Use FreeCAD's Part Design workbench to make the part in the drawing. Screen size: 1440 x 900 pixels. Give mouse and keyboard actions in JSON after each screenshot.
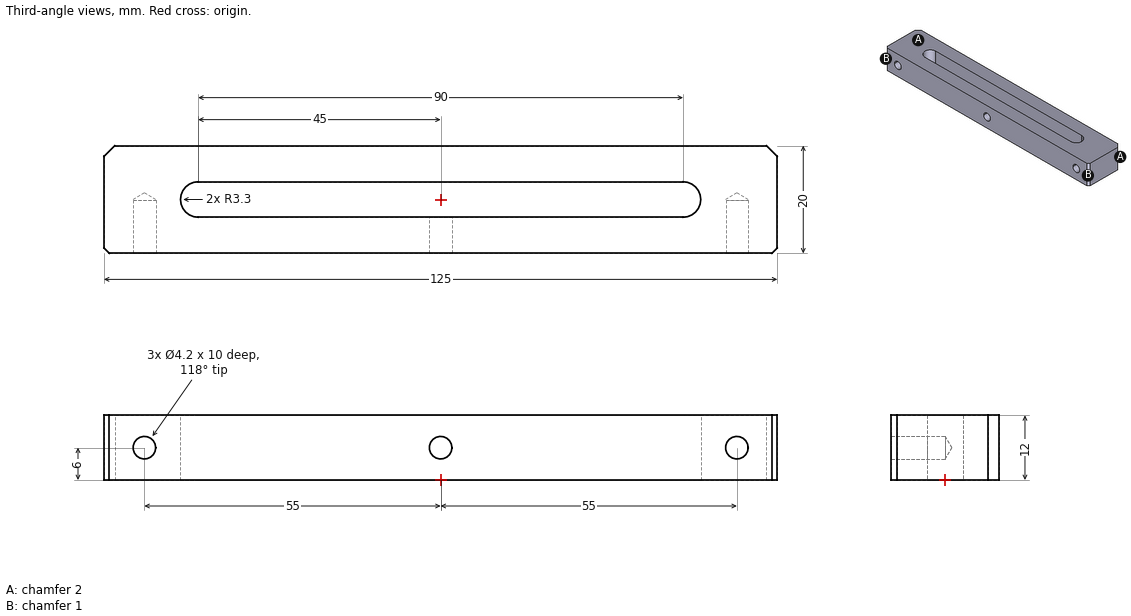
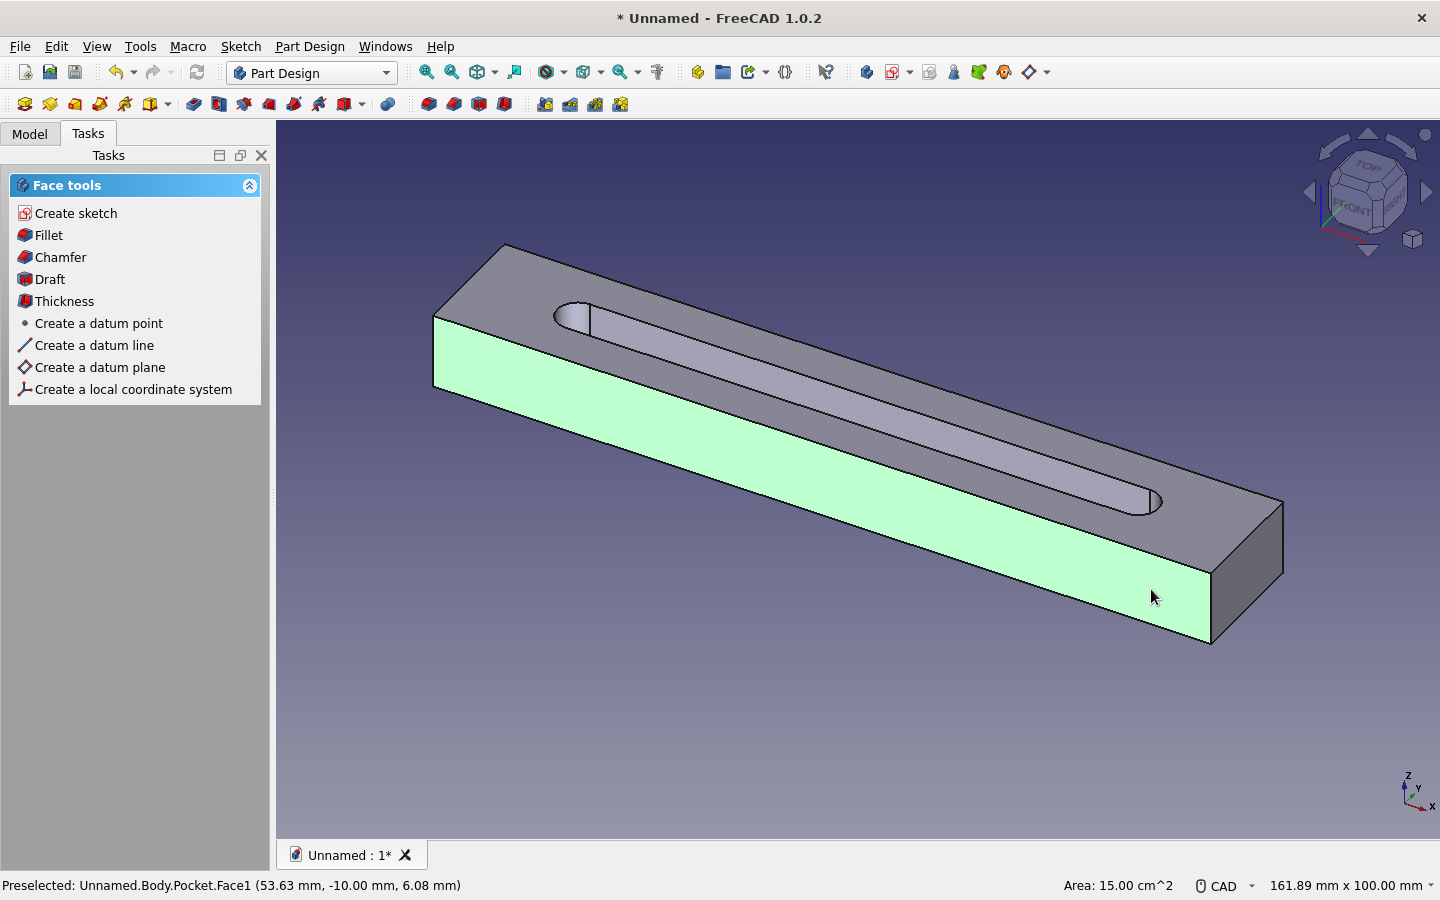
{"action": "left_click", "coordinate": [892, 72]}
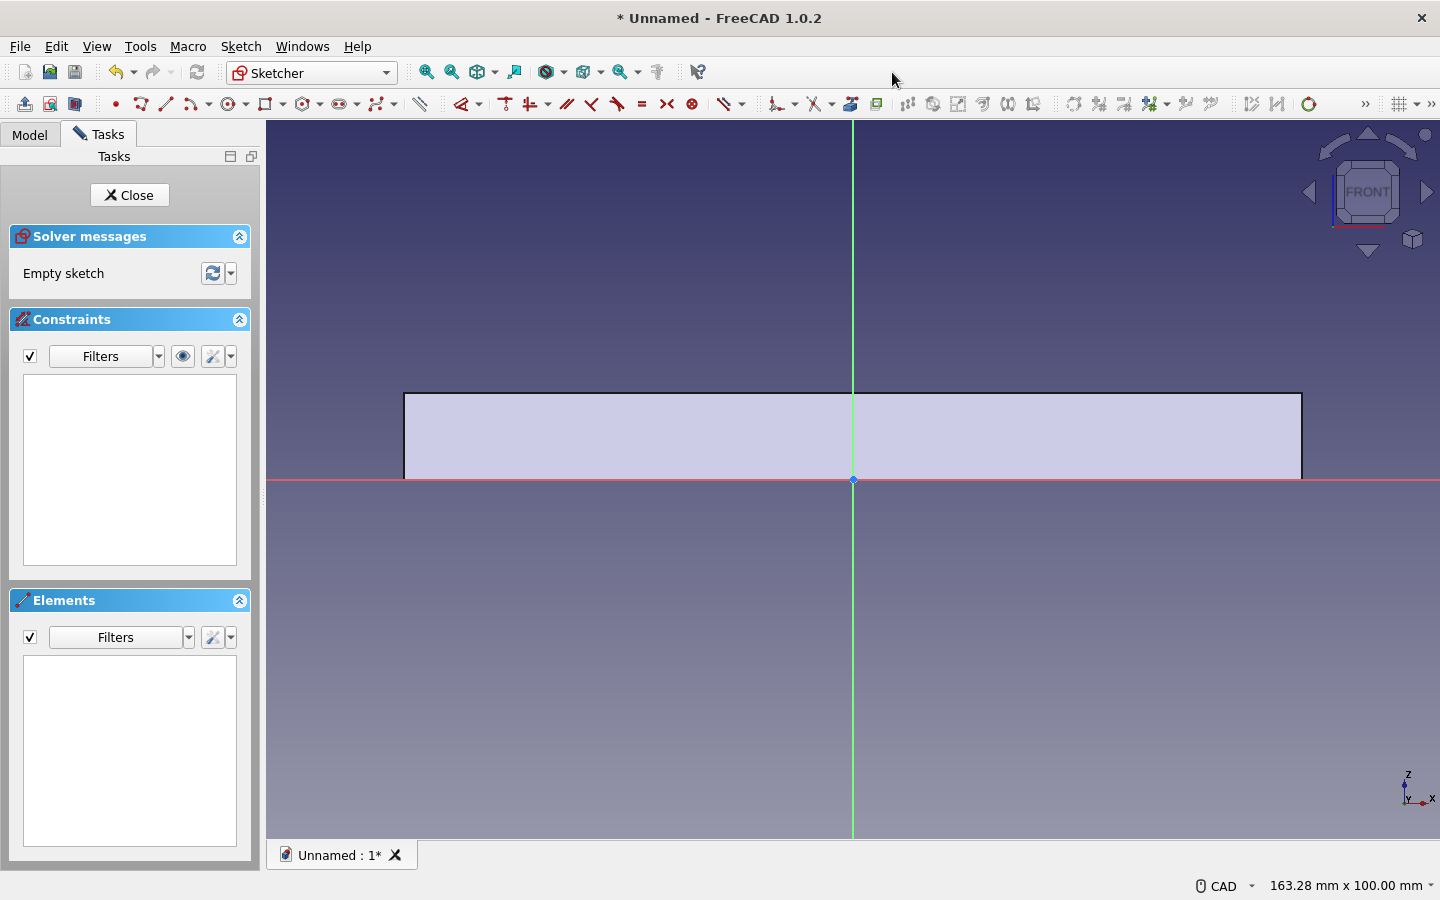
{"action": "scroll", "coordinate": [475, 611], "scroll_direction": "down", "scroll_amount": 1}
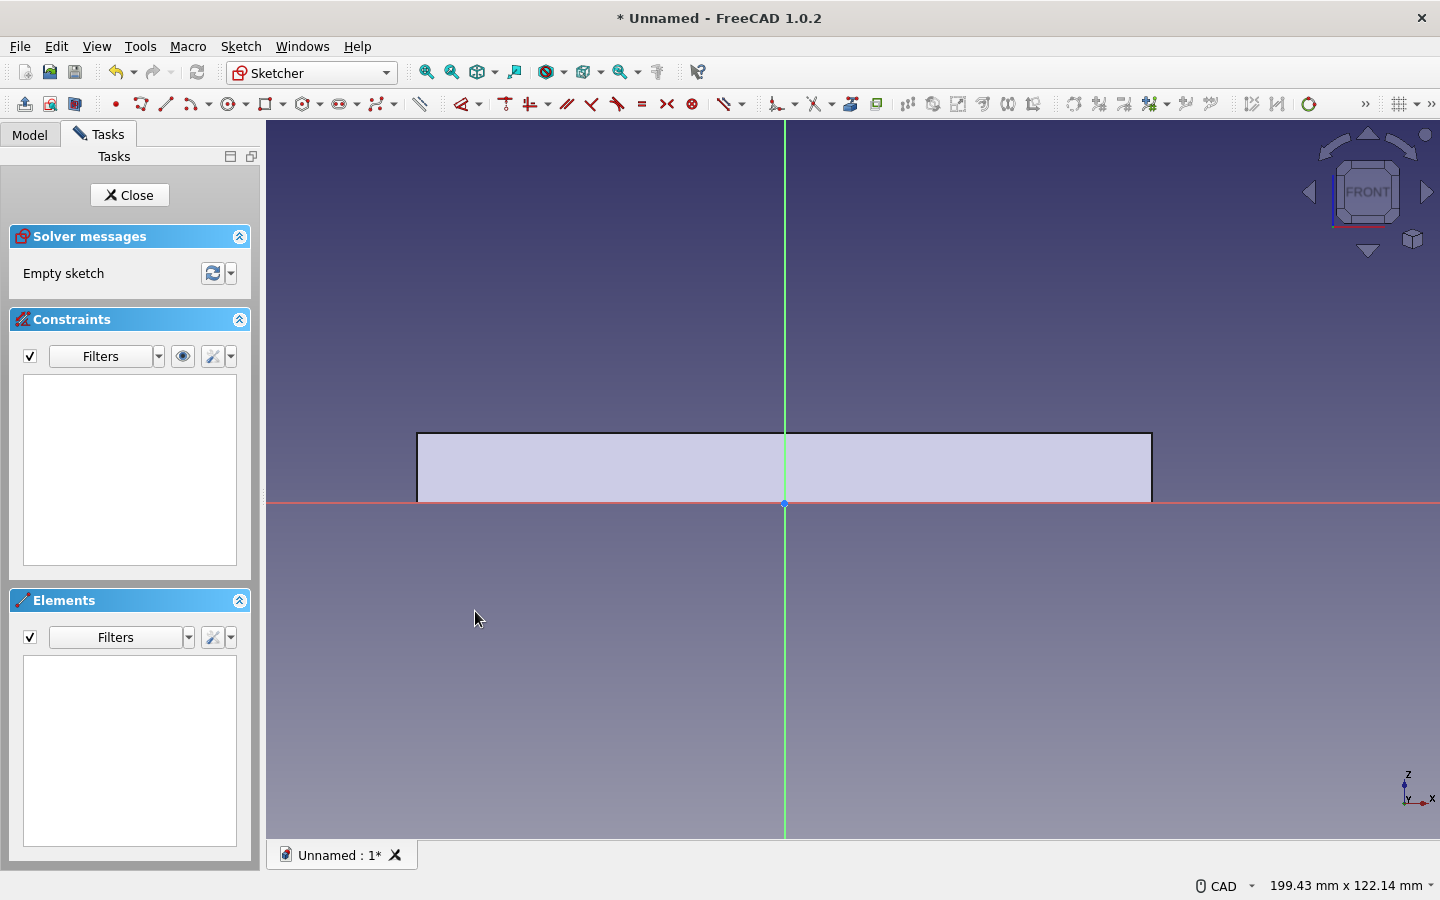
{"action": "key", "text": "g c"}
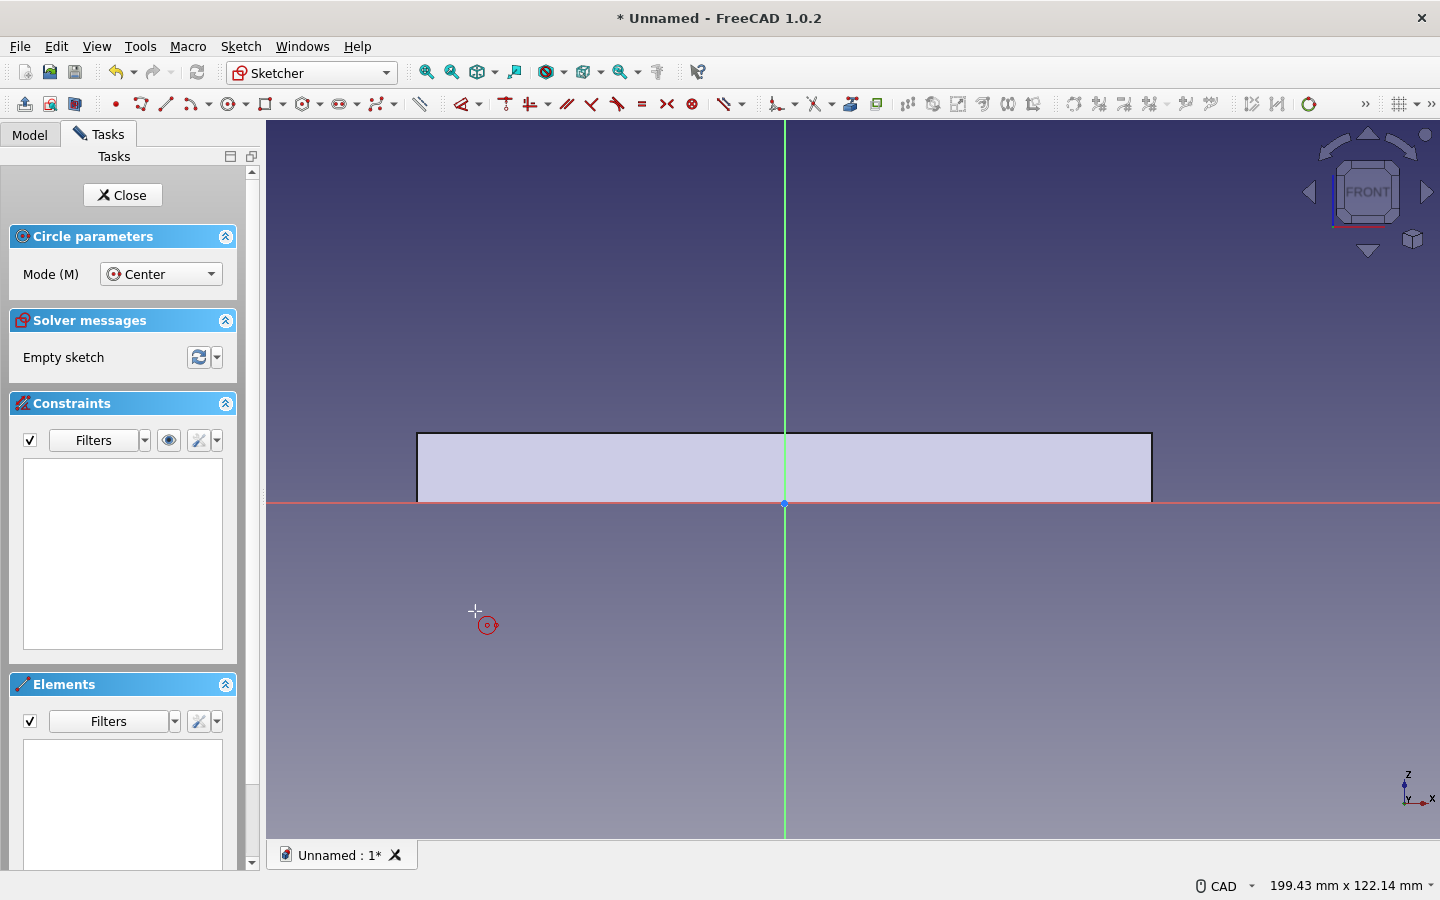
{"action": "scroll", "coordinate": [461, 468], "scroll_direction": "up", "scroll_amount": 4}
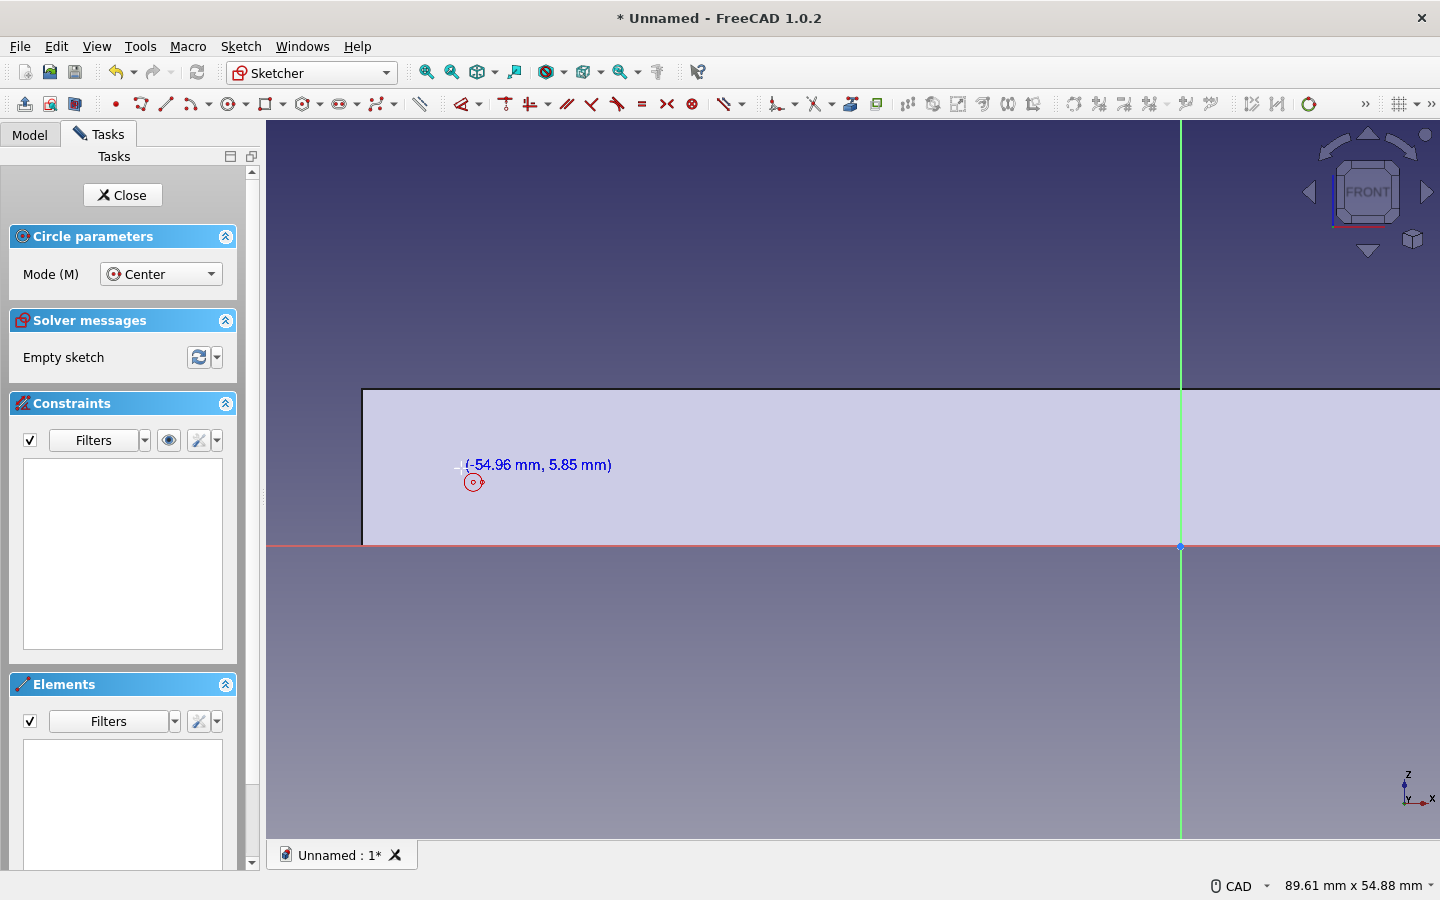
{"action": "left_click", "coordinate": [460, 468]}
{"action": "mouse_move", "coordinate": [480, 448]}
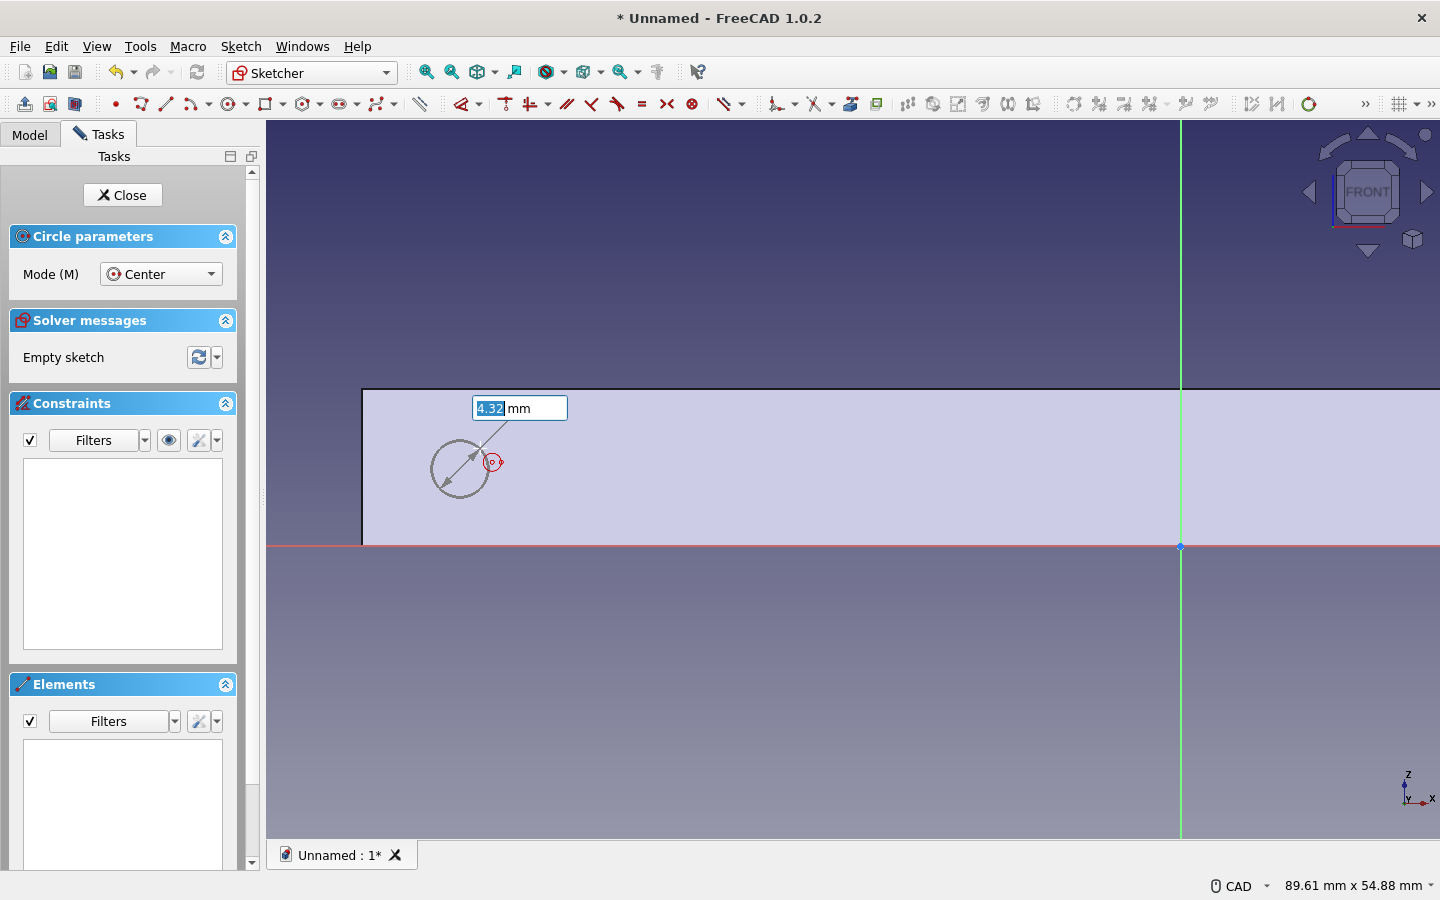
{"action": "type", "text": "4.2"}
{"action": "key", "text": "Return"}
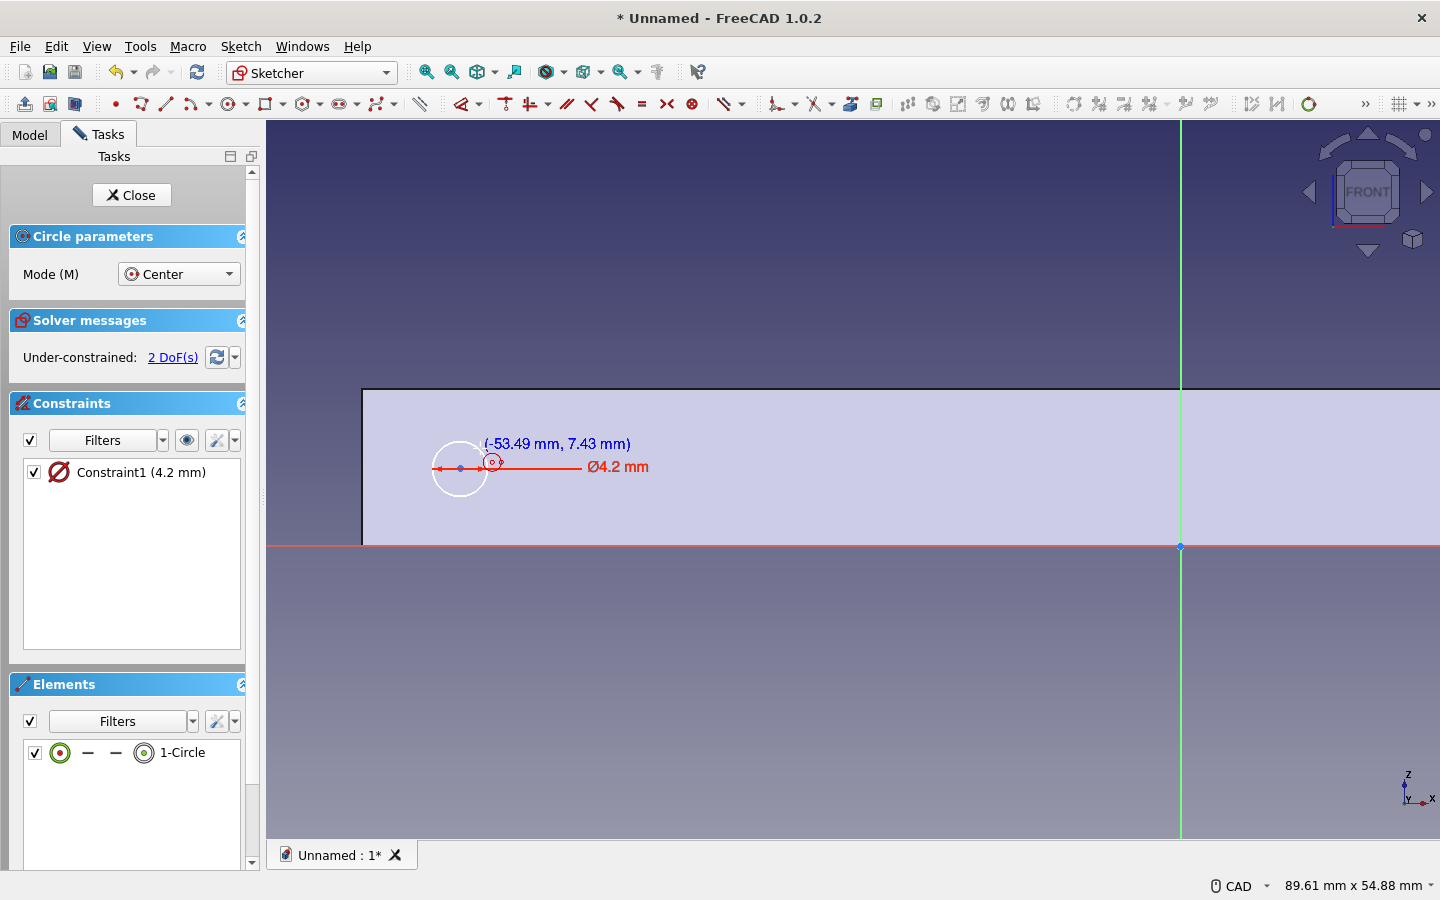
{"action": "left_click", "coordinate": [1181, 468]}
{"action": "mouse_move", "coordinate": [1200, 448]}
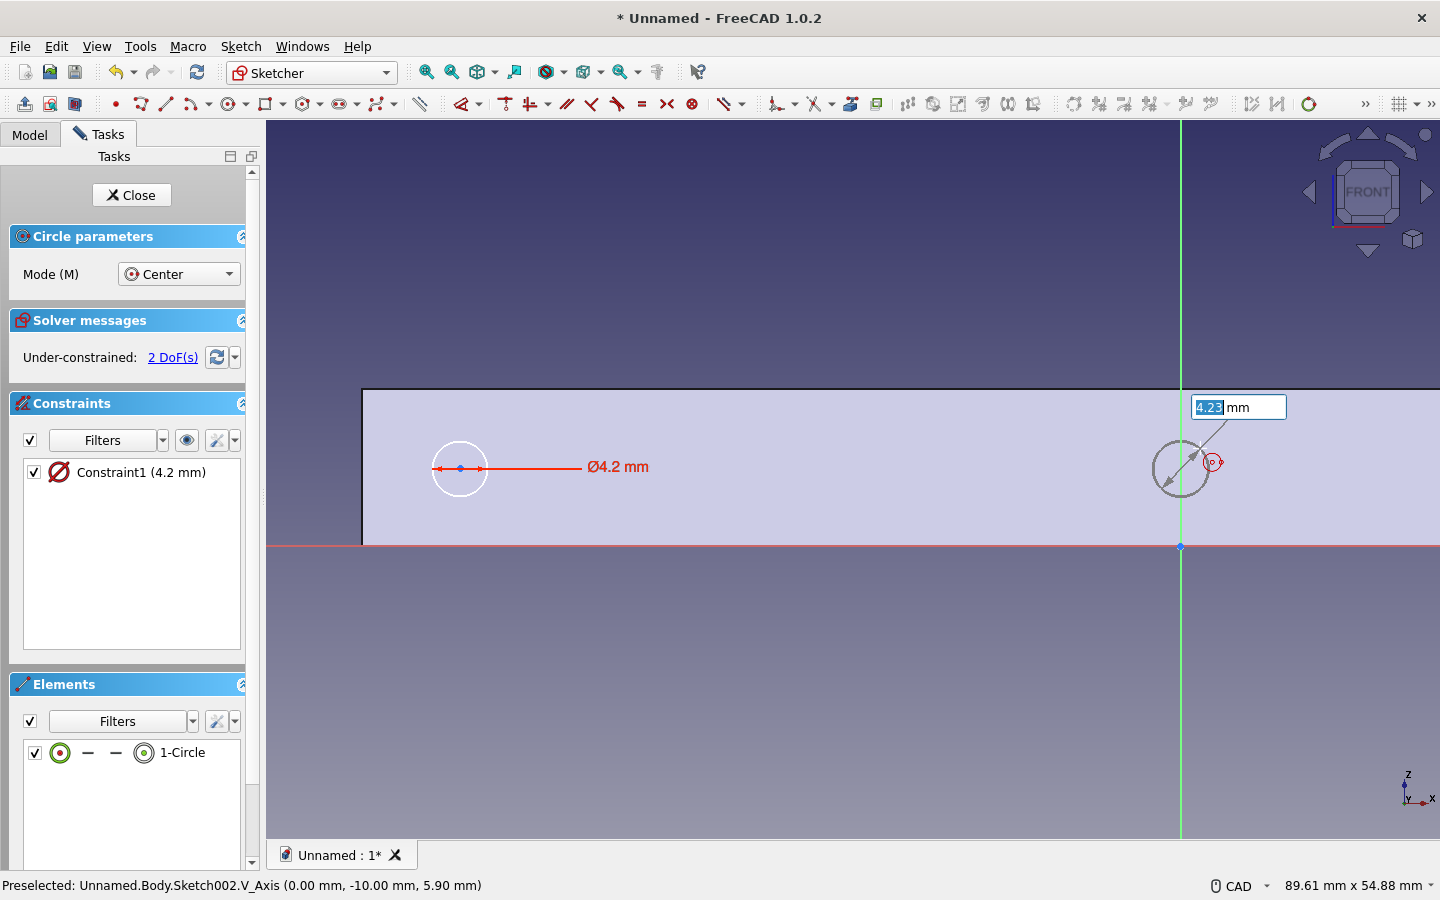
{"action": "type", "text": "4.2"}
{"action": "key", "text": "Return"}